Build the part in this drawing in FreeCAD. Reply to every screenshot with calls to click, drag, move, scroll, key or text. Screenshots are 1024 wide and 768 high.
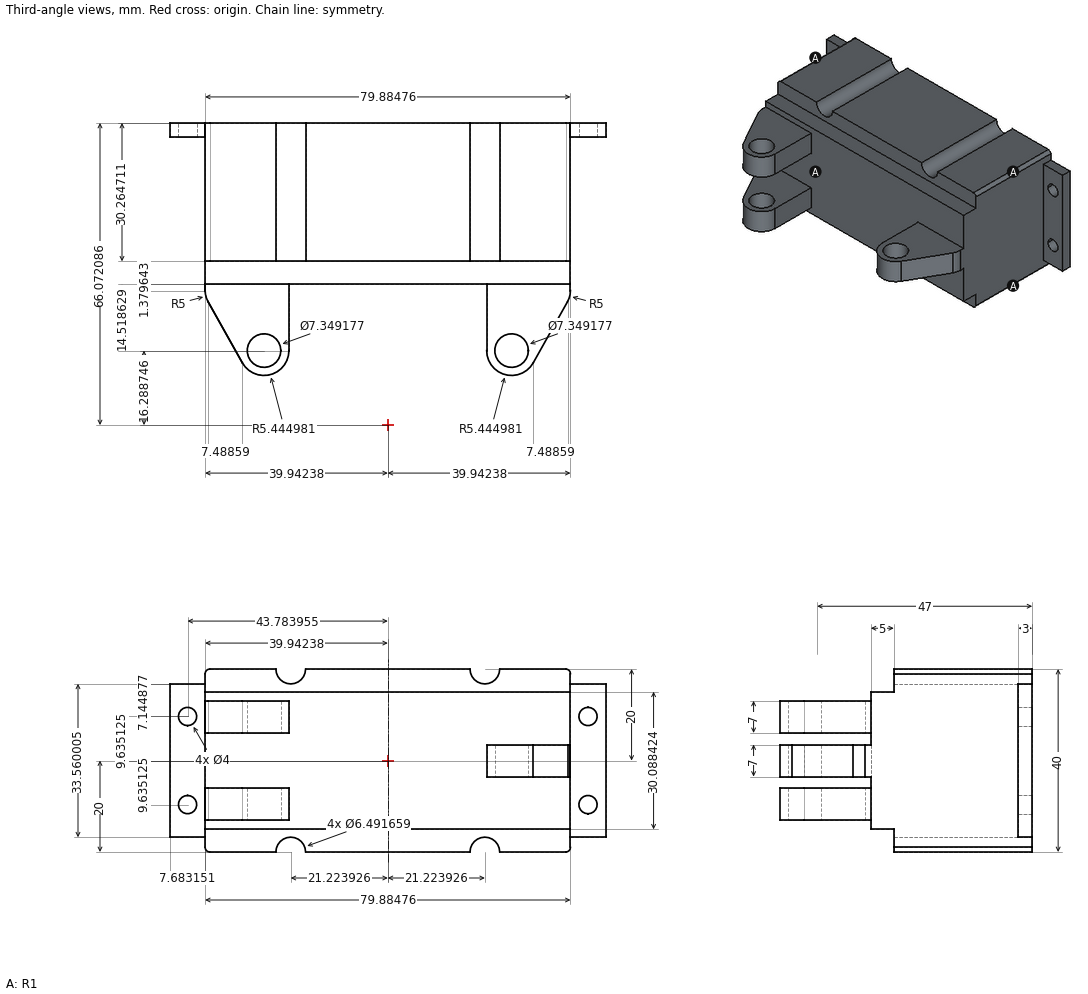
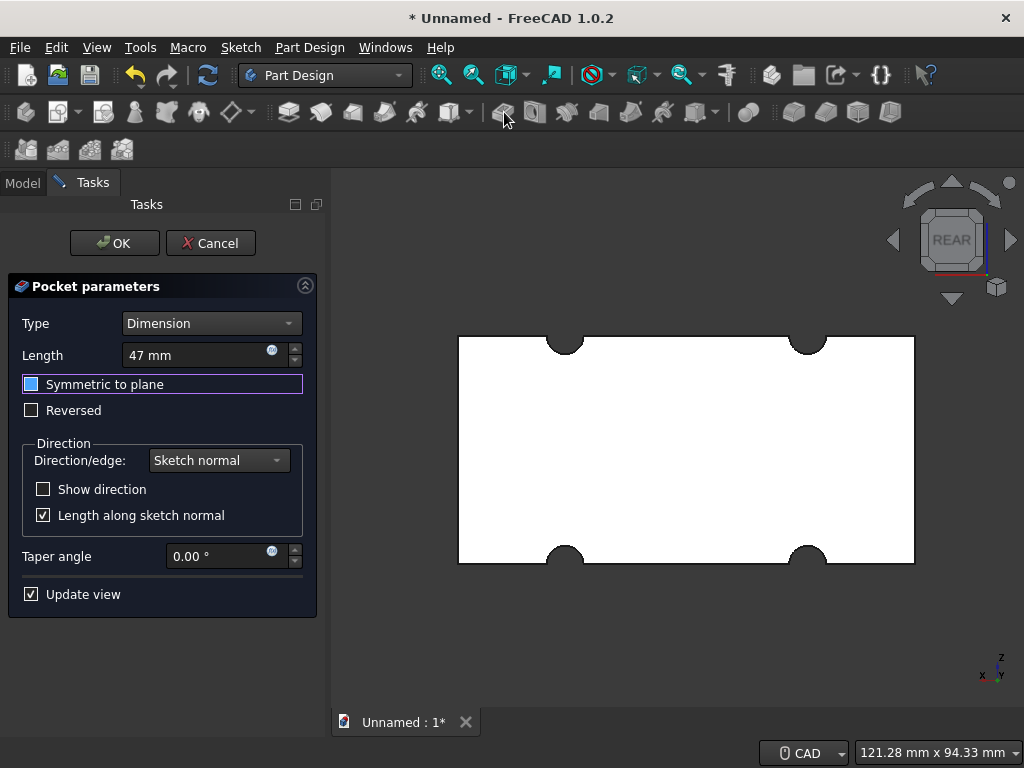
click(115, 243)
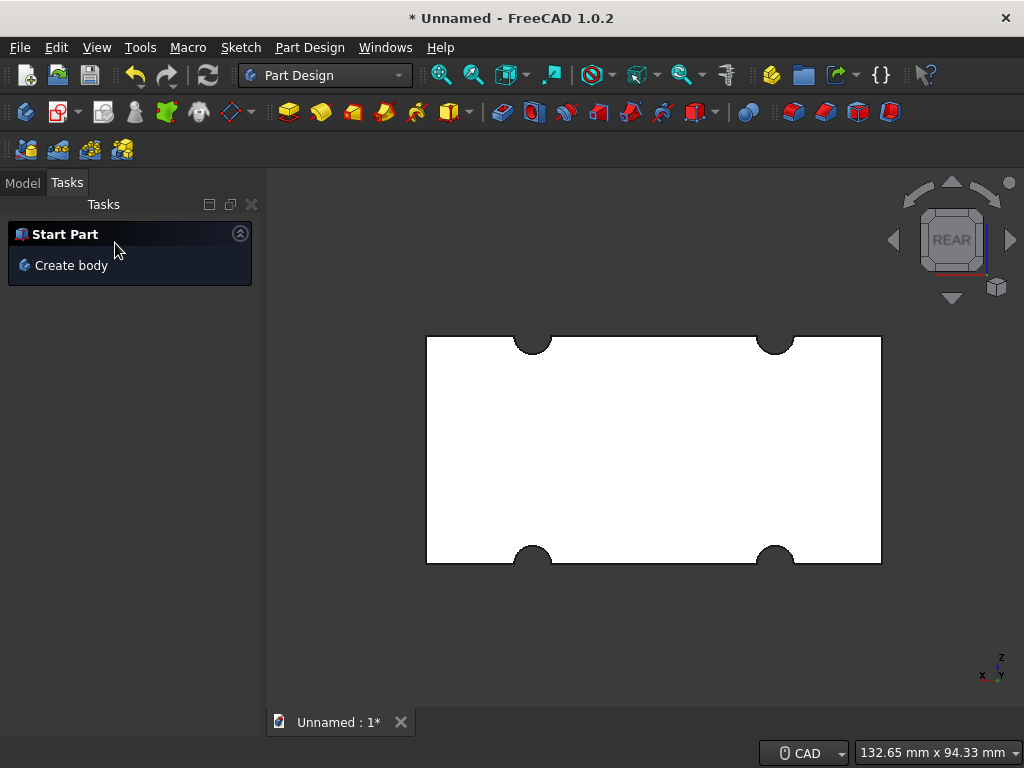
key(0)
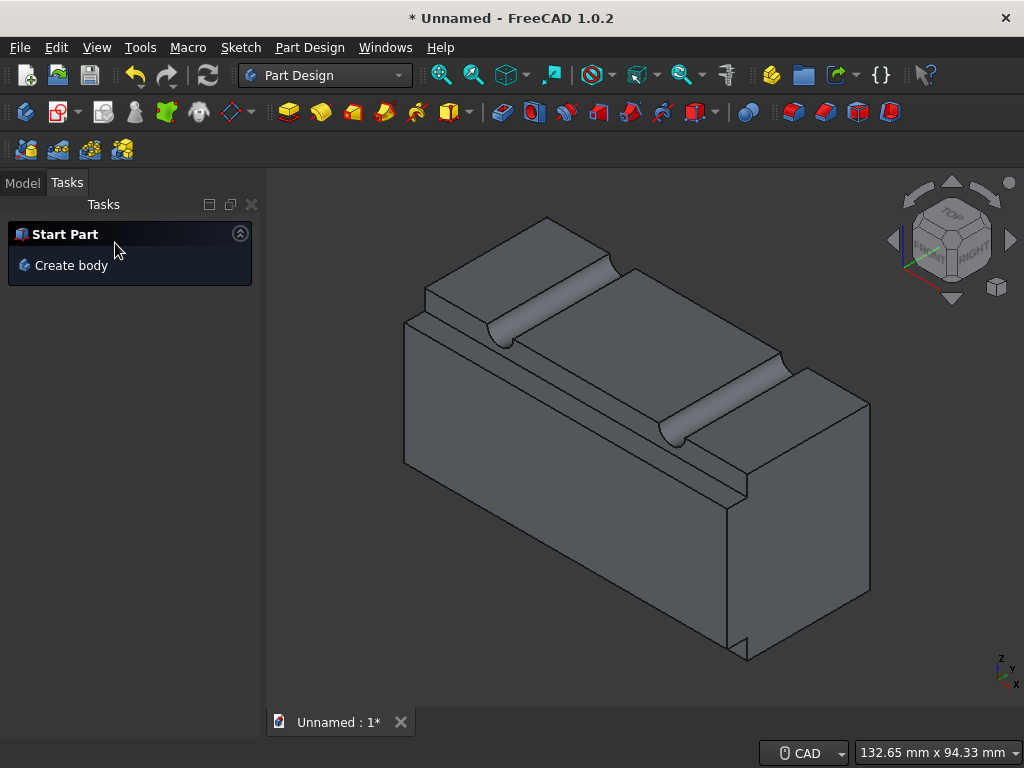
click(809, 438)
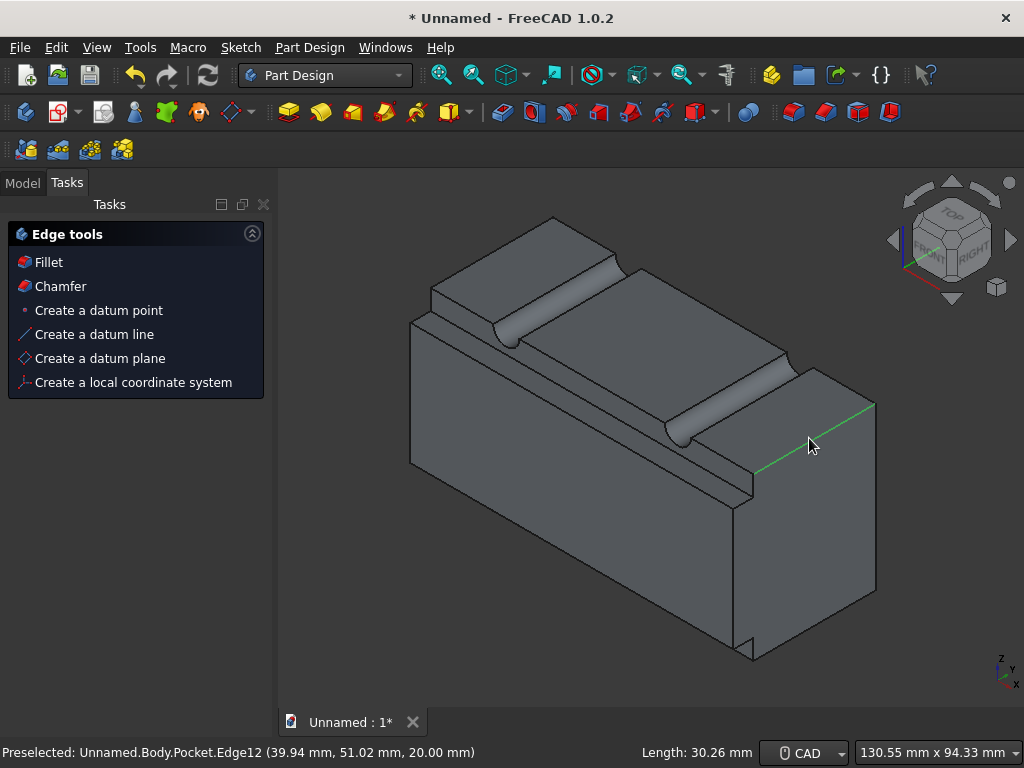
key(2)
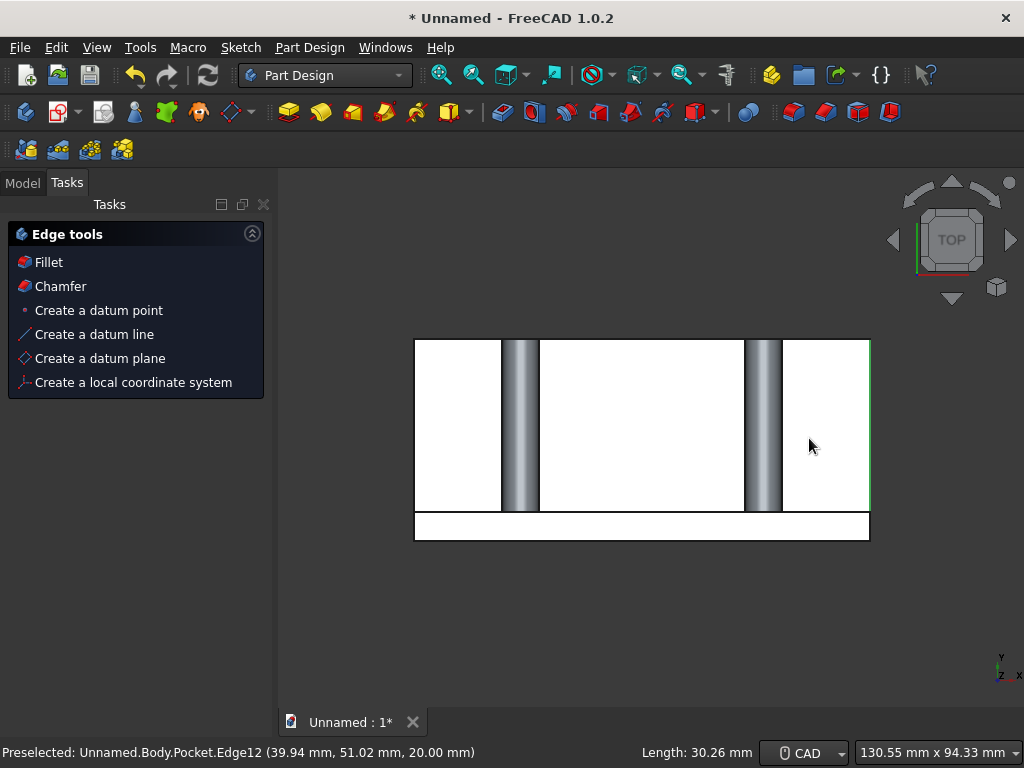
click(414, 424, ctrl)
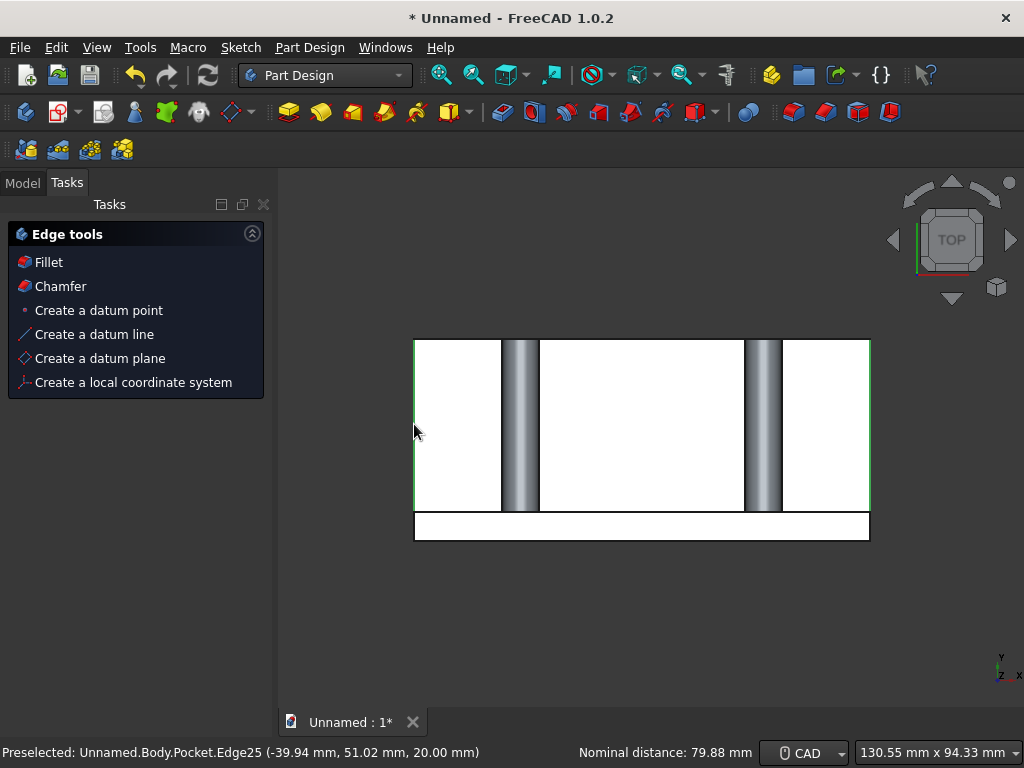
key(1)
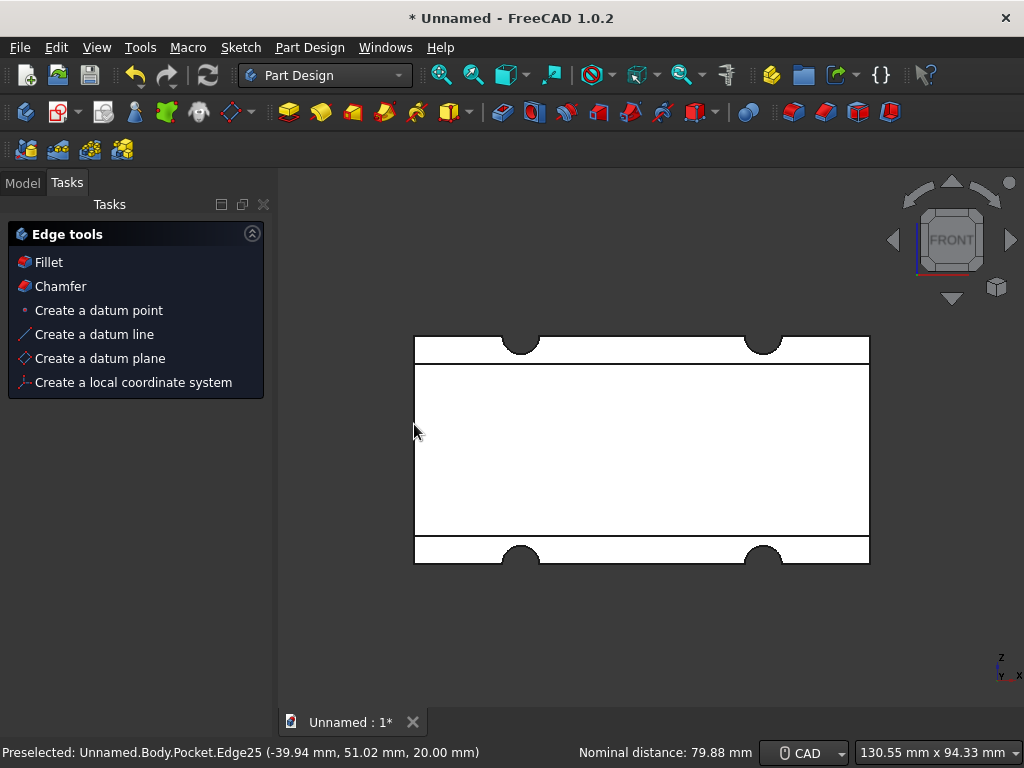
key(3)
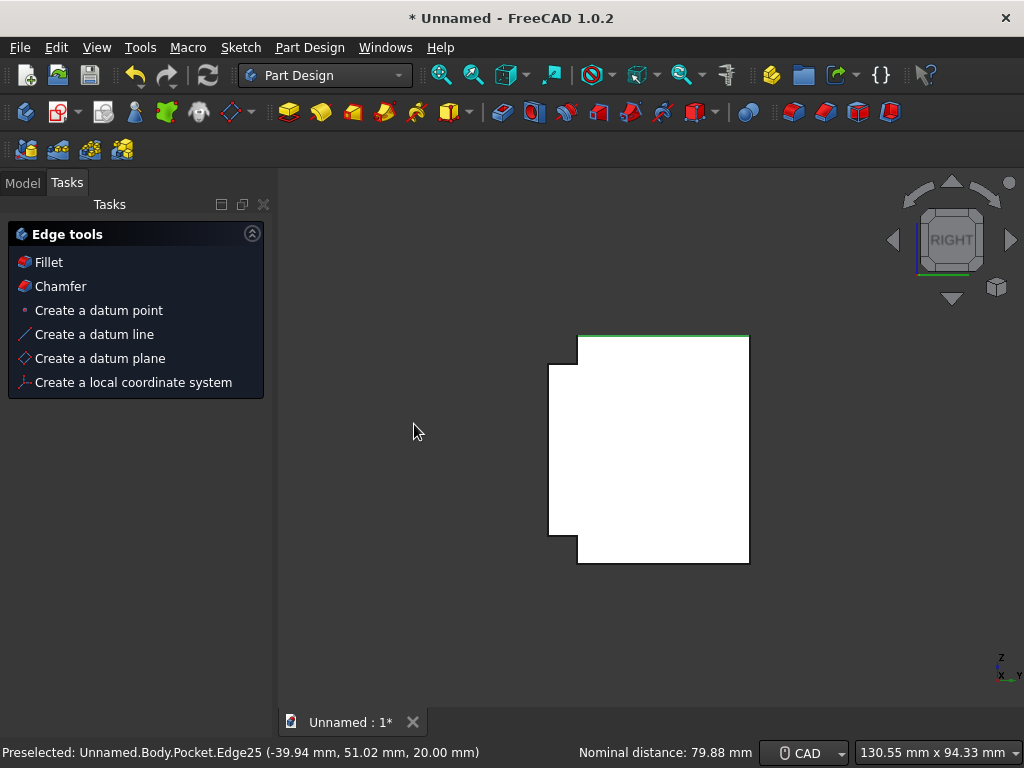
click(442, 76)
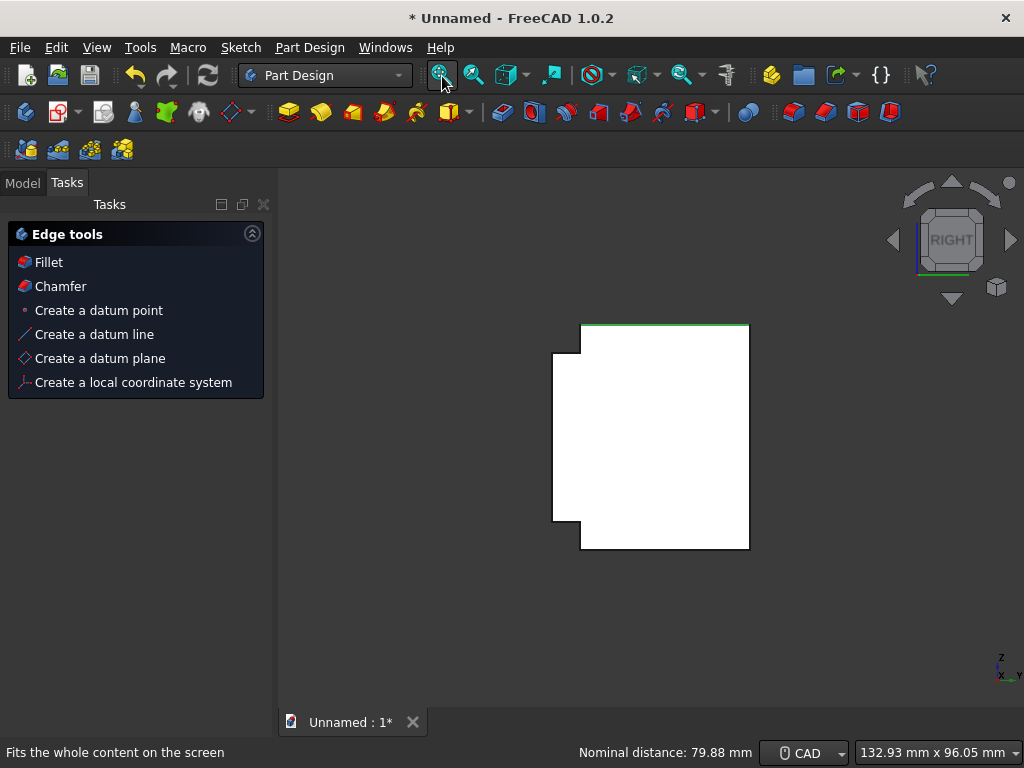
click(665, 549, ctrl)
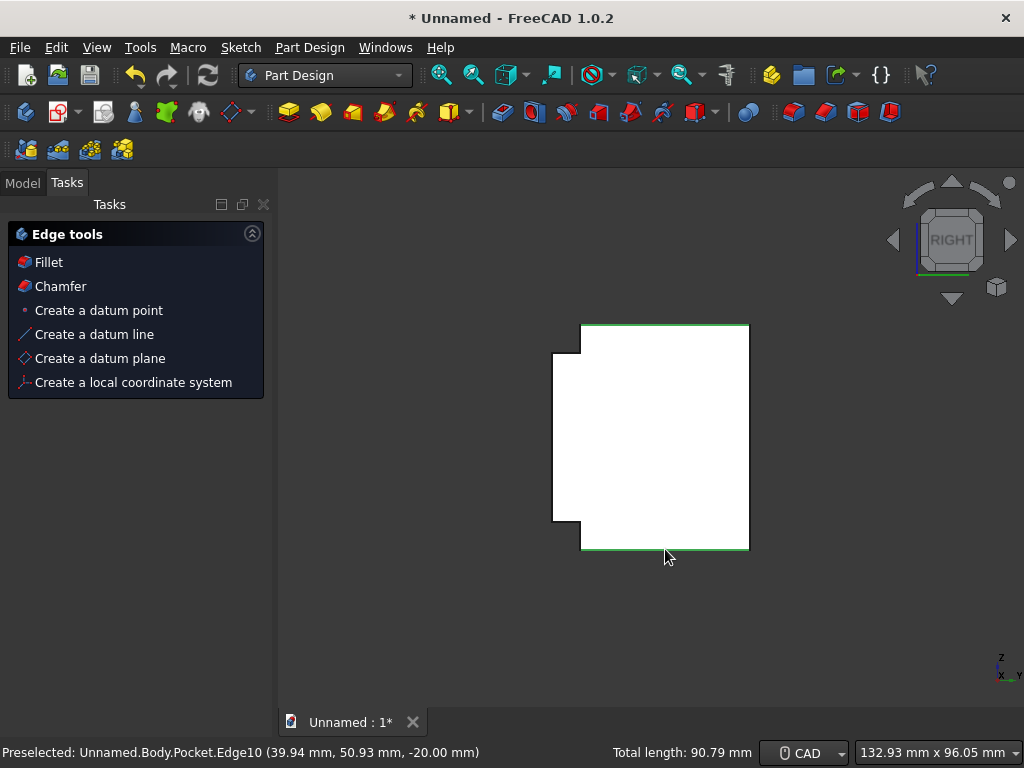
key(5)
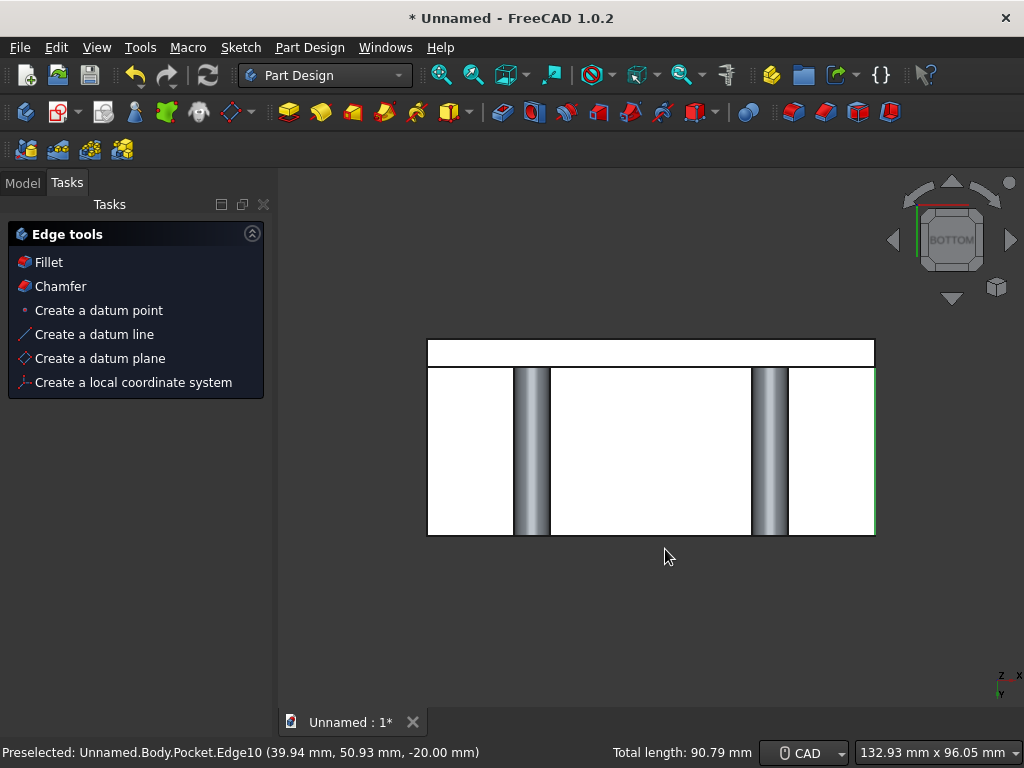
click(427, 451, ctrl)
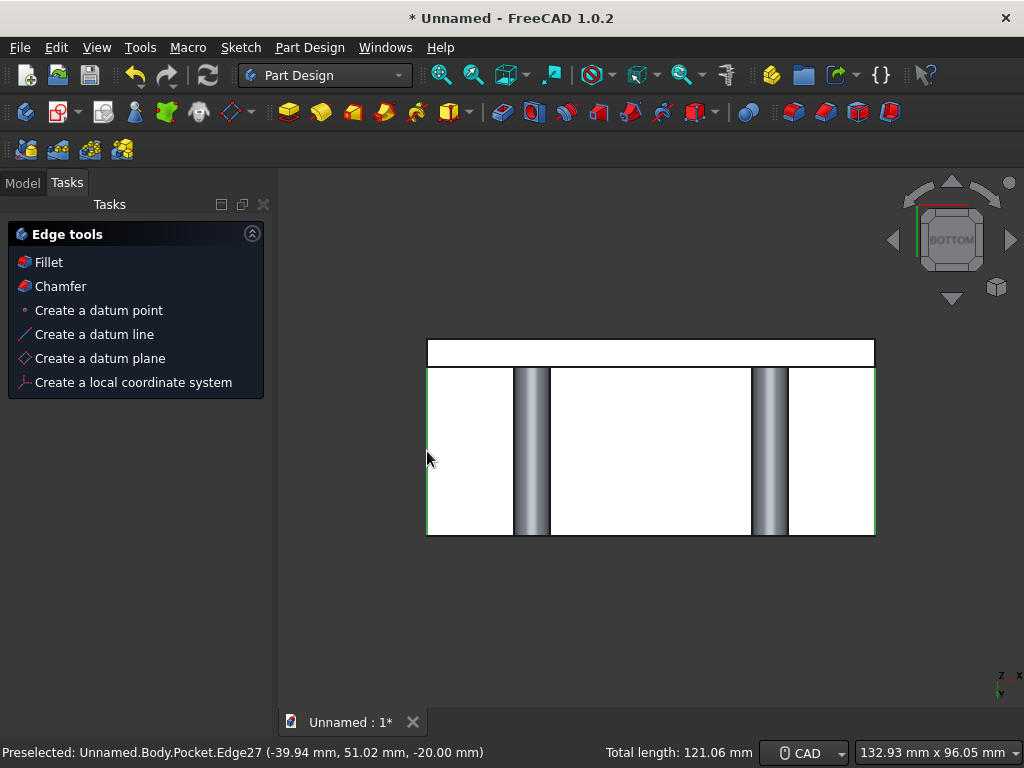
click(794, 112)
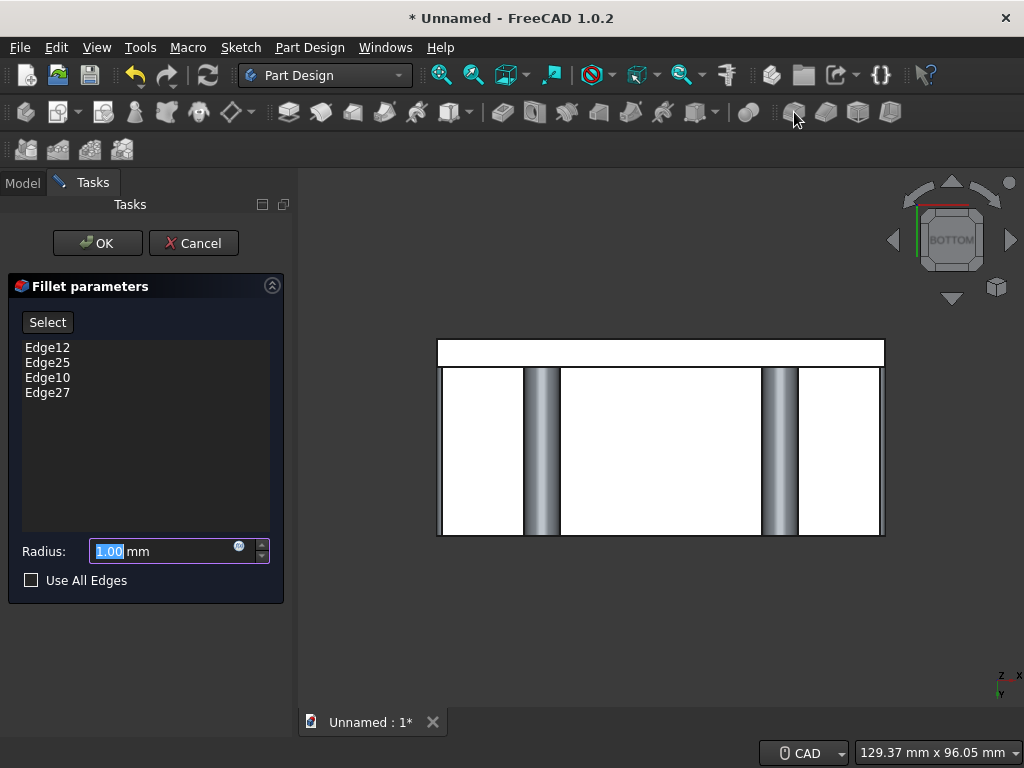
text(1)
key(Tab)